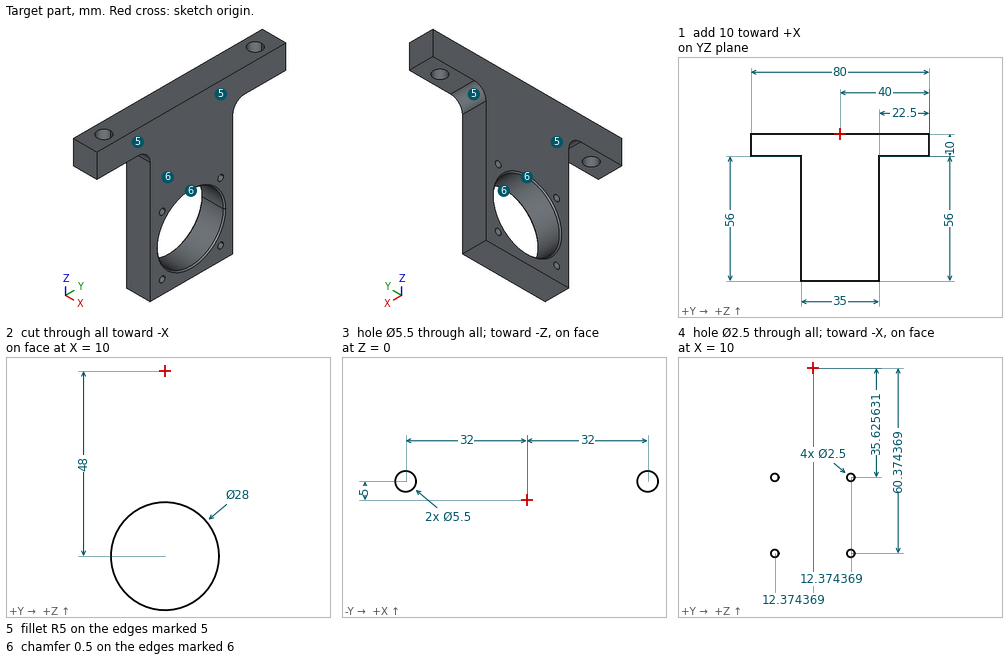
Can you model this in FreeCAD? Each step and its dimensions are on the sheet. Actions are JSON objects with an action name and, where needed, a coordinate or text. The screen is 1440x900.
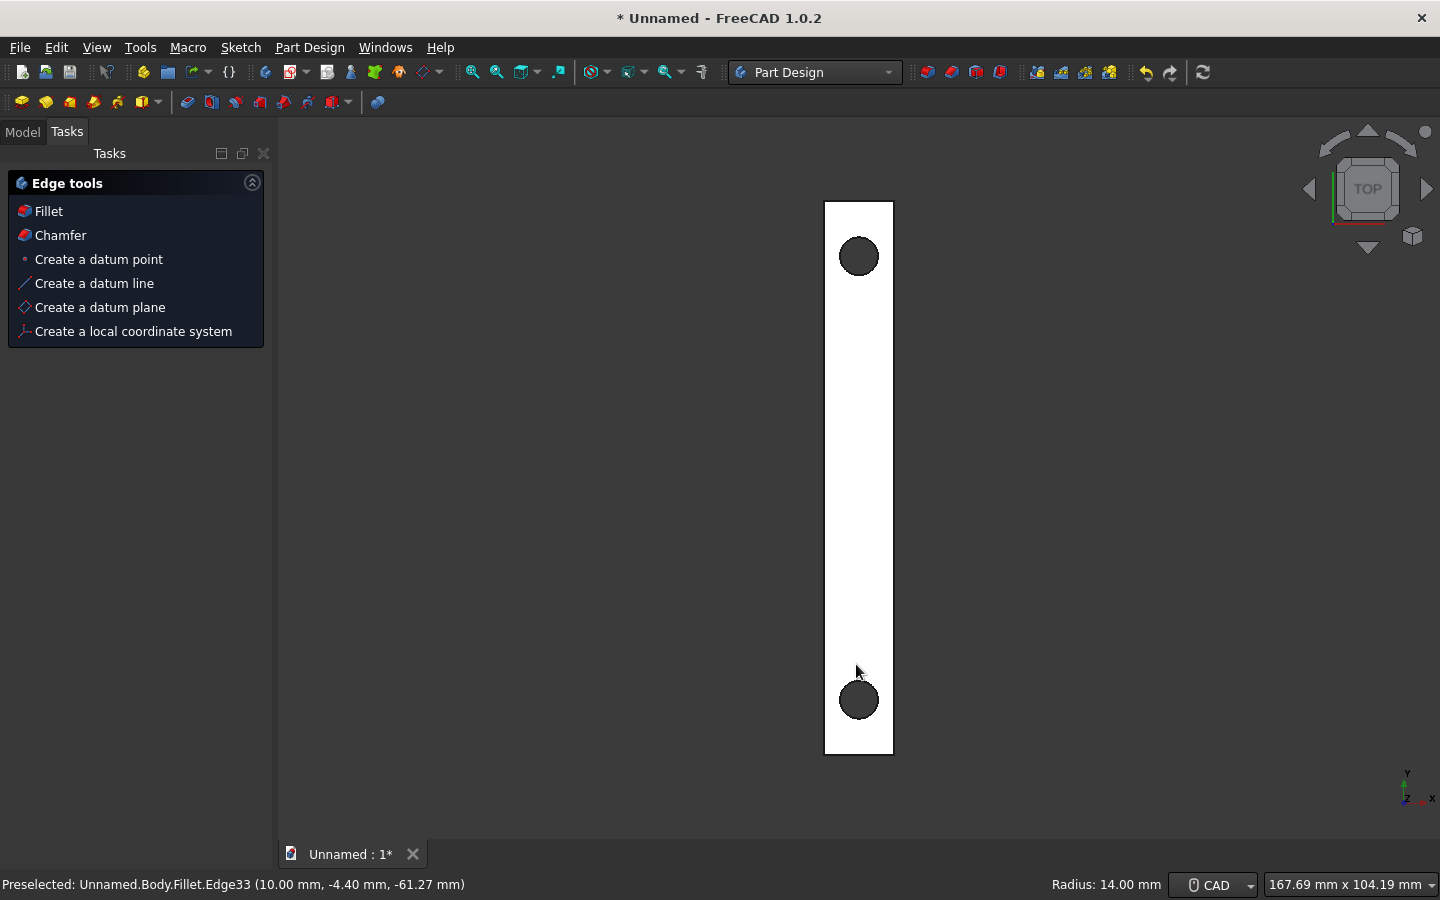
{"action": "key", "text": "0"}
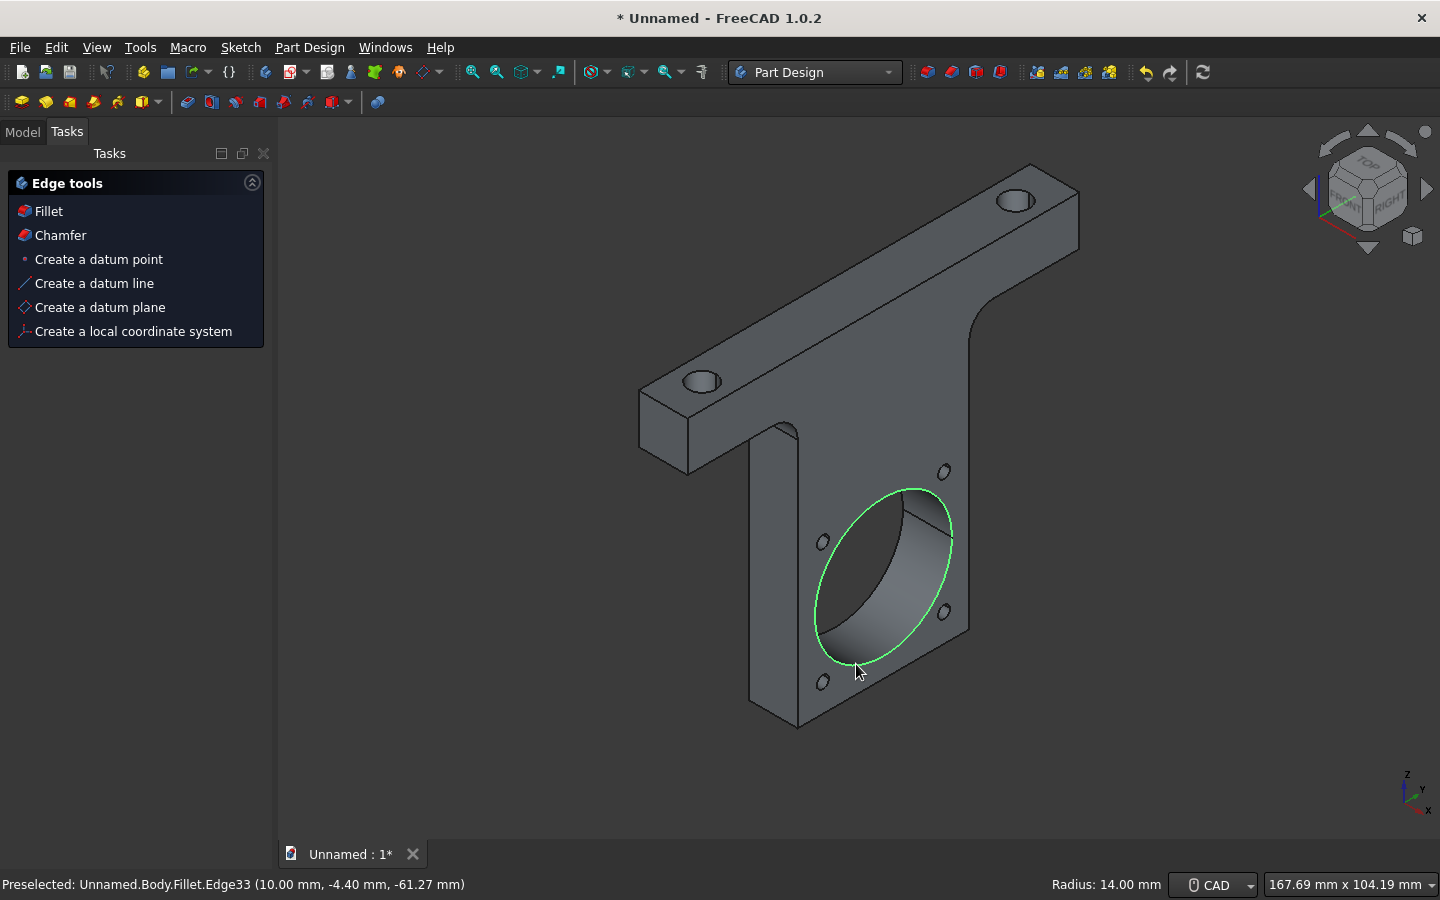
{"action": "key", "text": "1"}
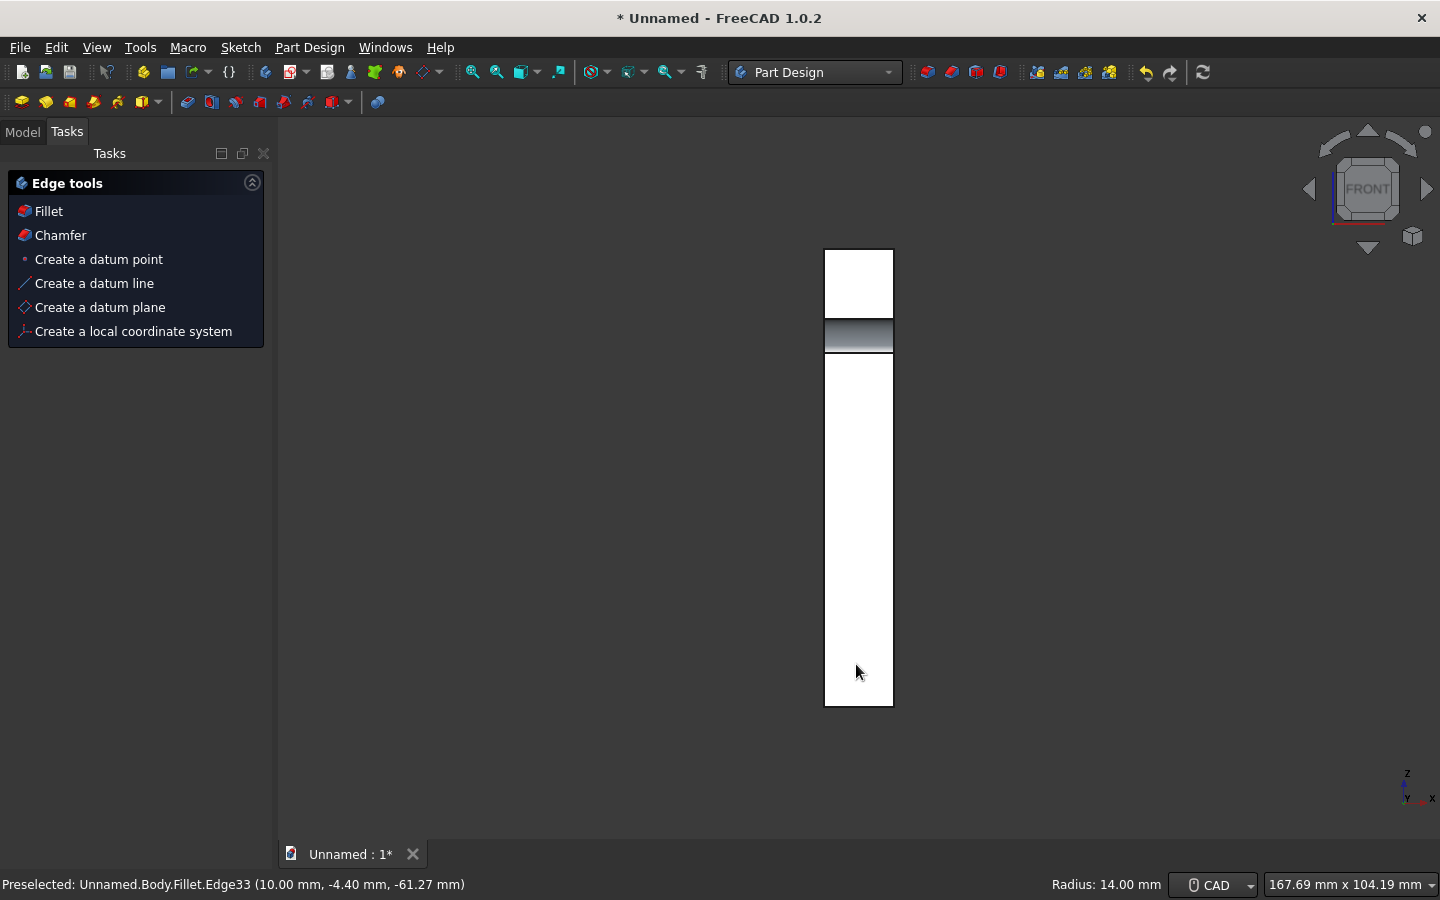
{"action": "key", "text": "3"}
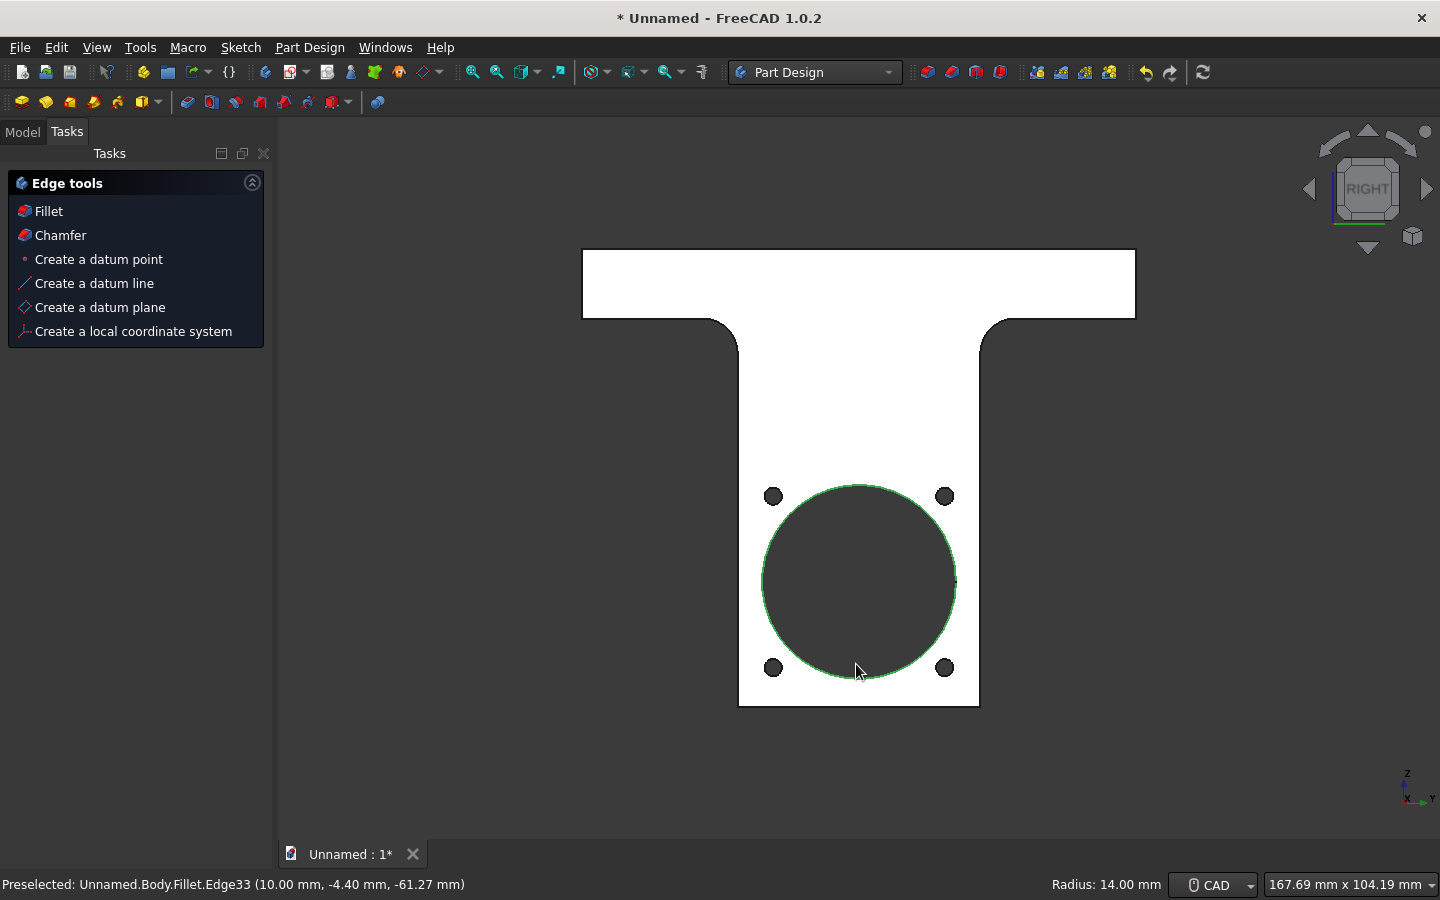
{"action": "key", "text": "5"}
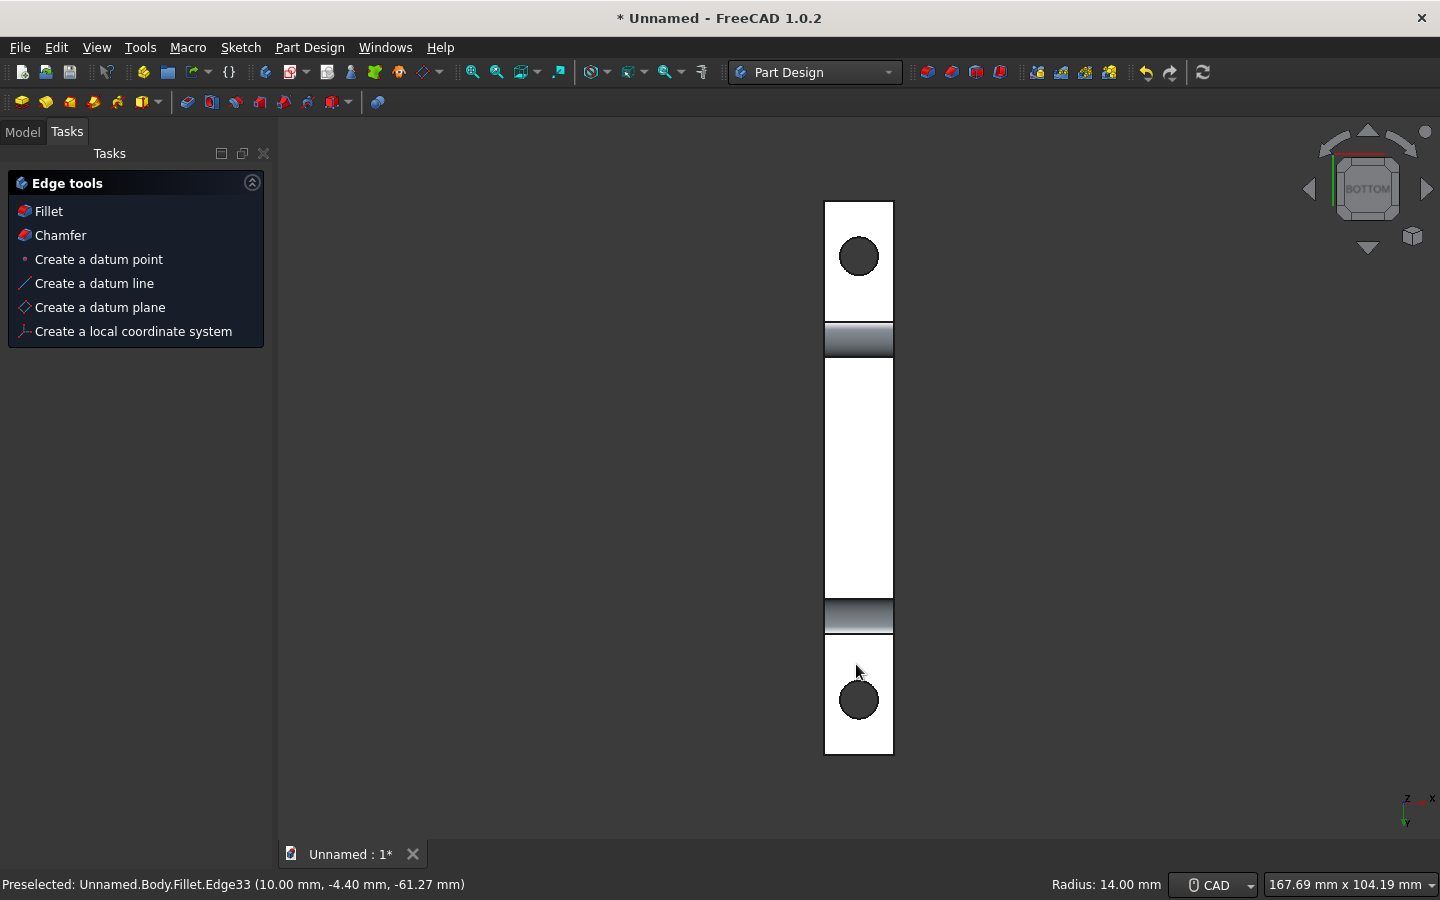
{"action": "key", "text": "4"}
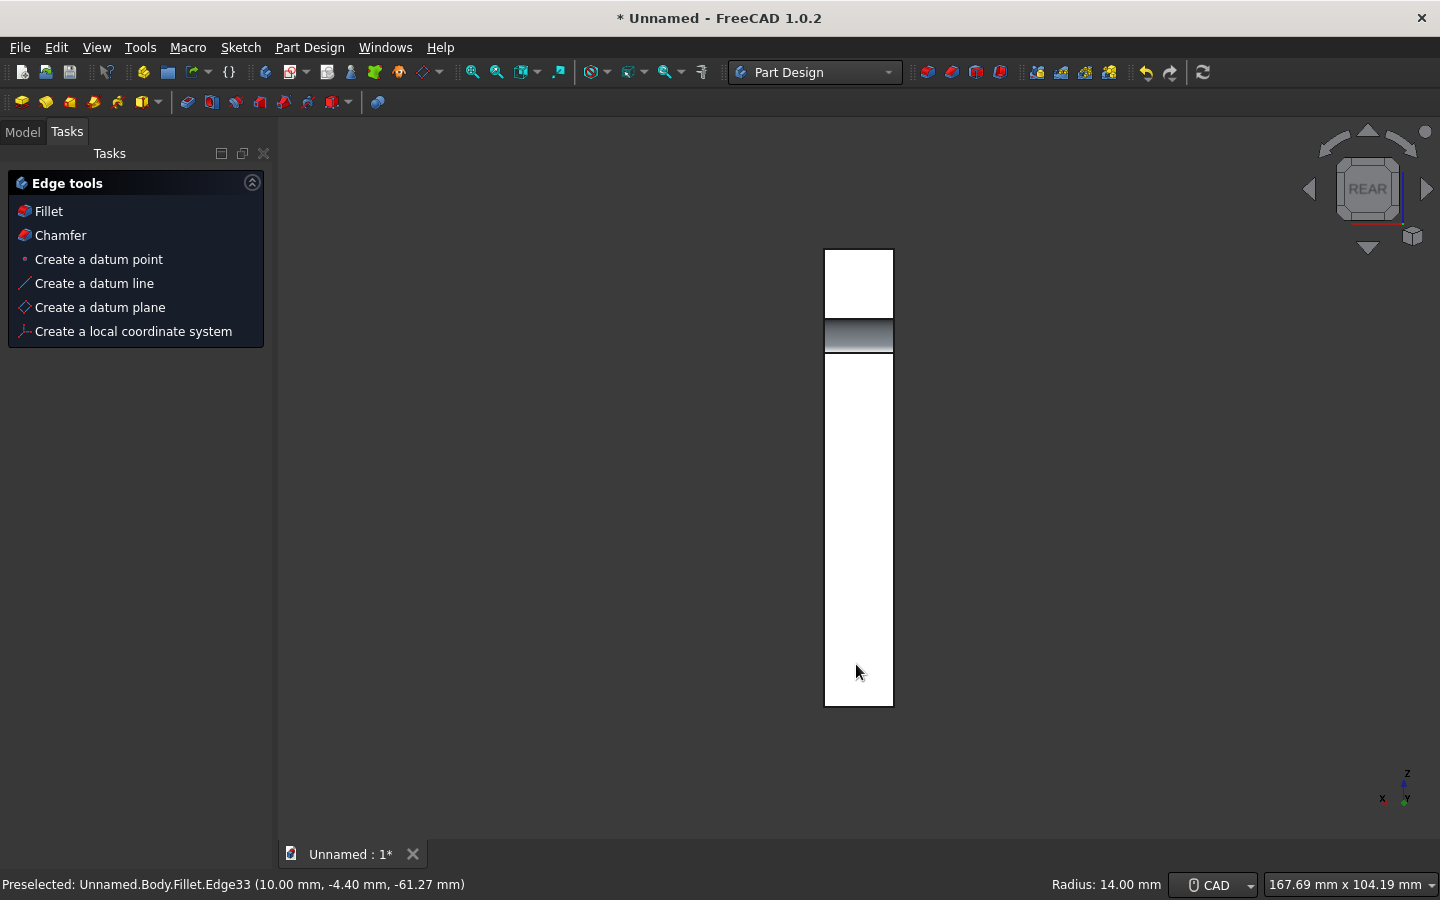
{"action": "key", "text": "6"}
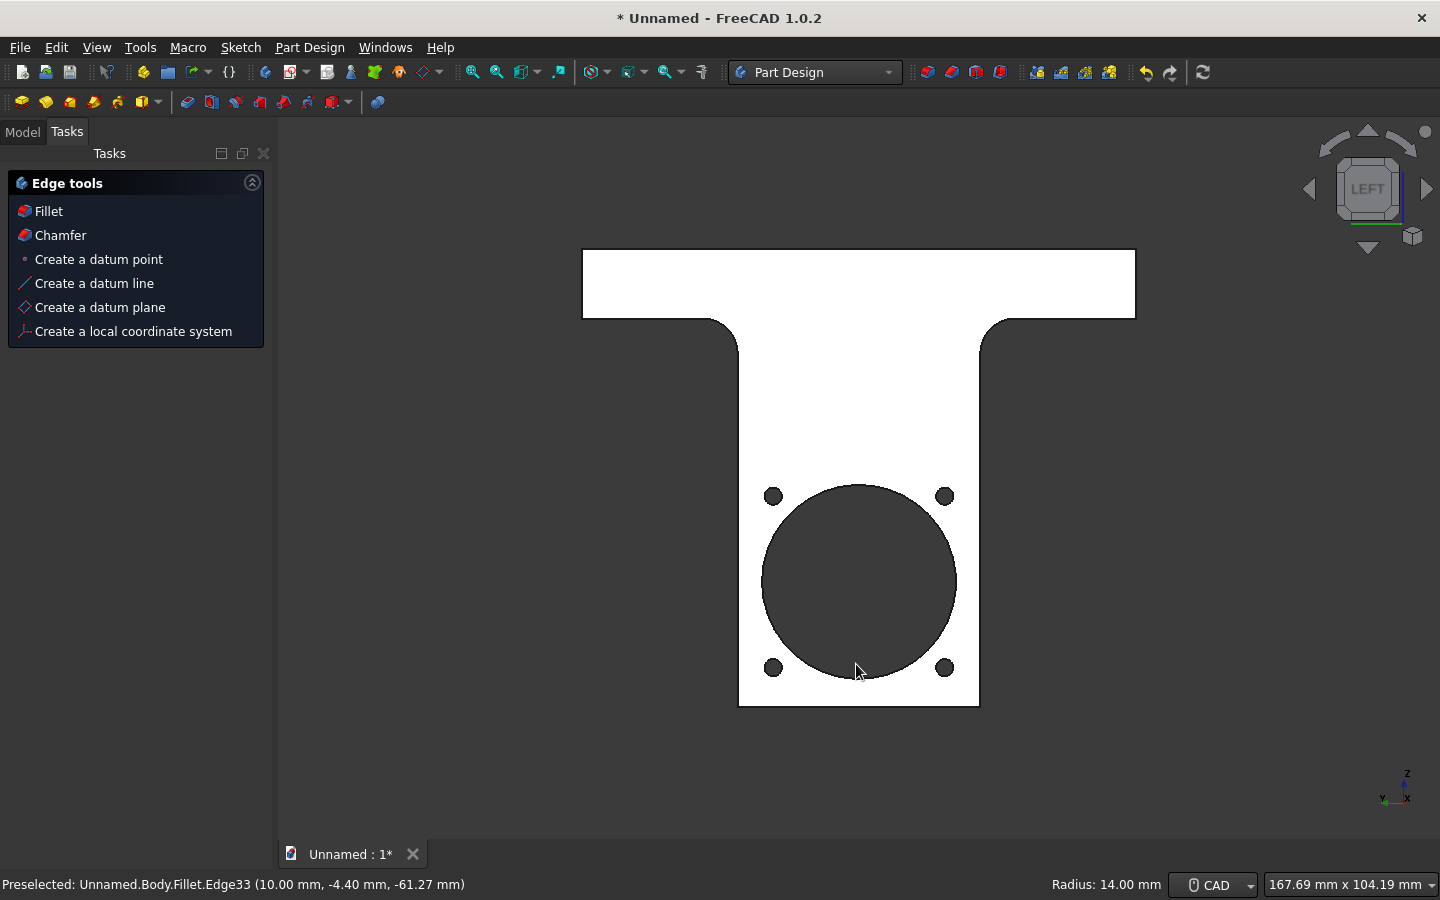
{"action": "left_click", "coordinate": [829, 489], "text": "ctrl"}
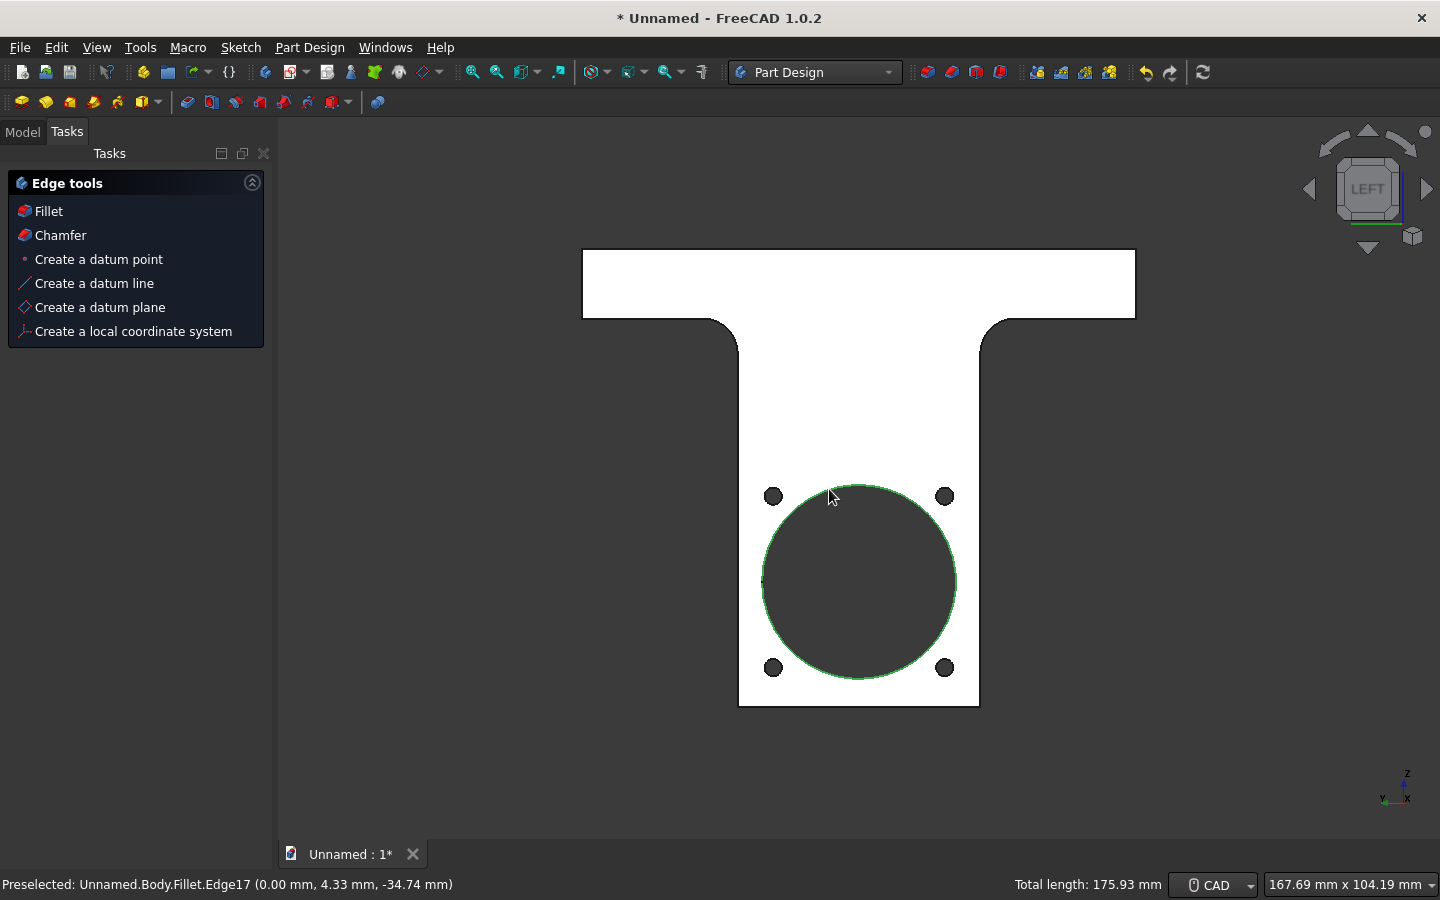
{"action": "left_click", "coordinate": [952, 72]}